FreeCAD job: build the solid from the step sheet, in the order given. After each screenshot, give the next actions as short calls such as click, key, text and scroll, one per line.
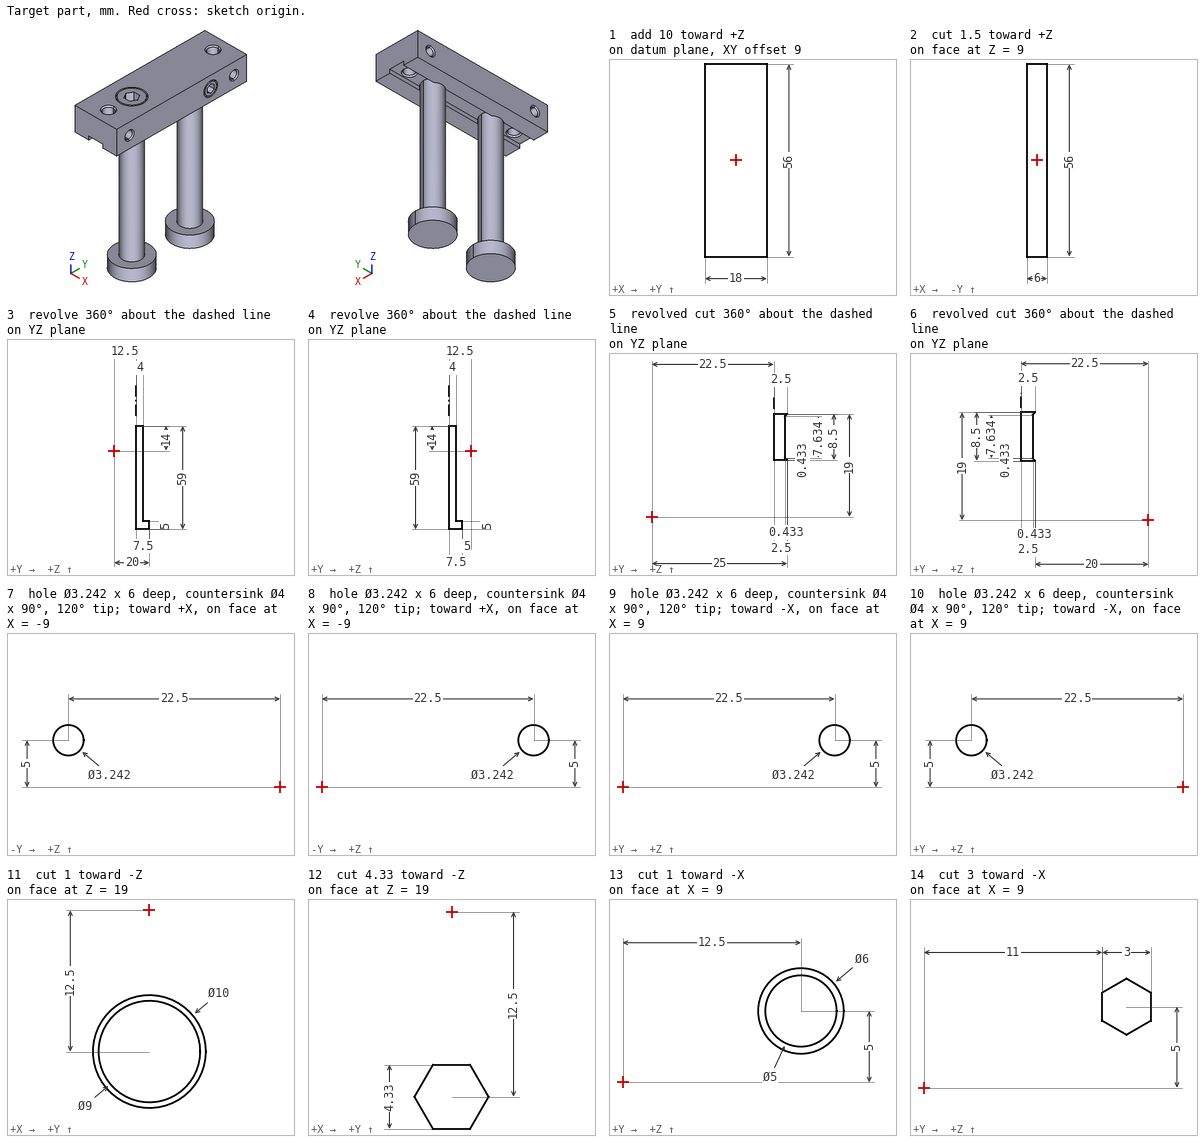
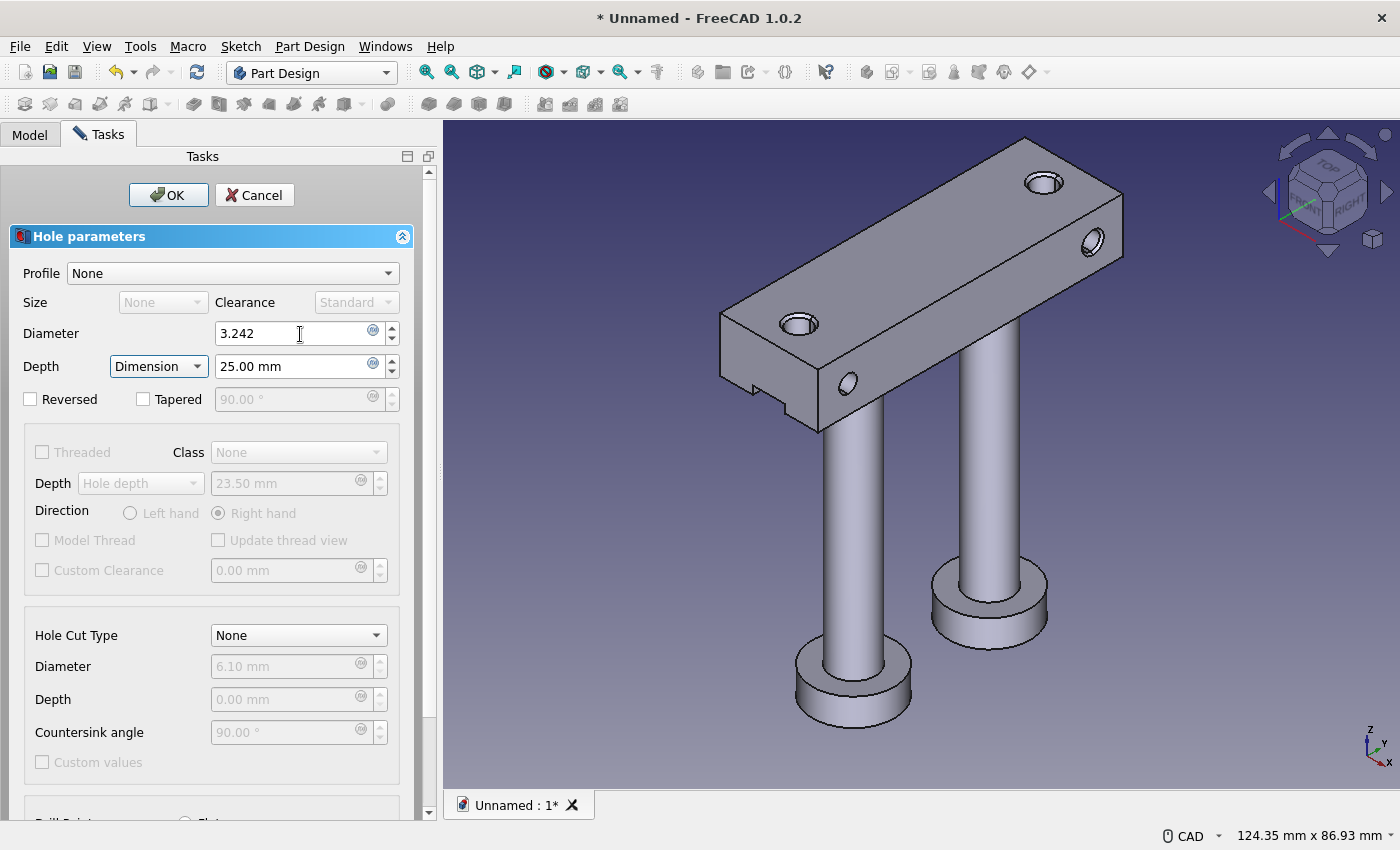
triple_click(300, 366)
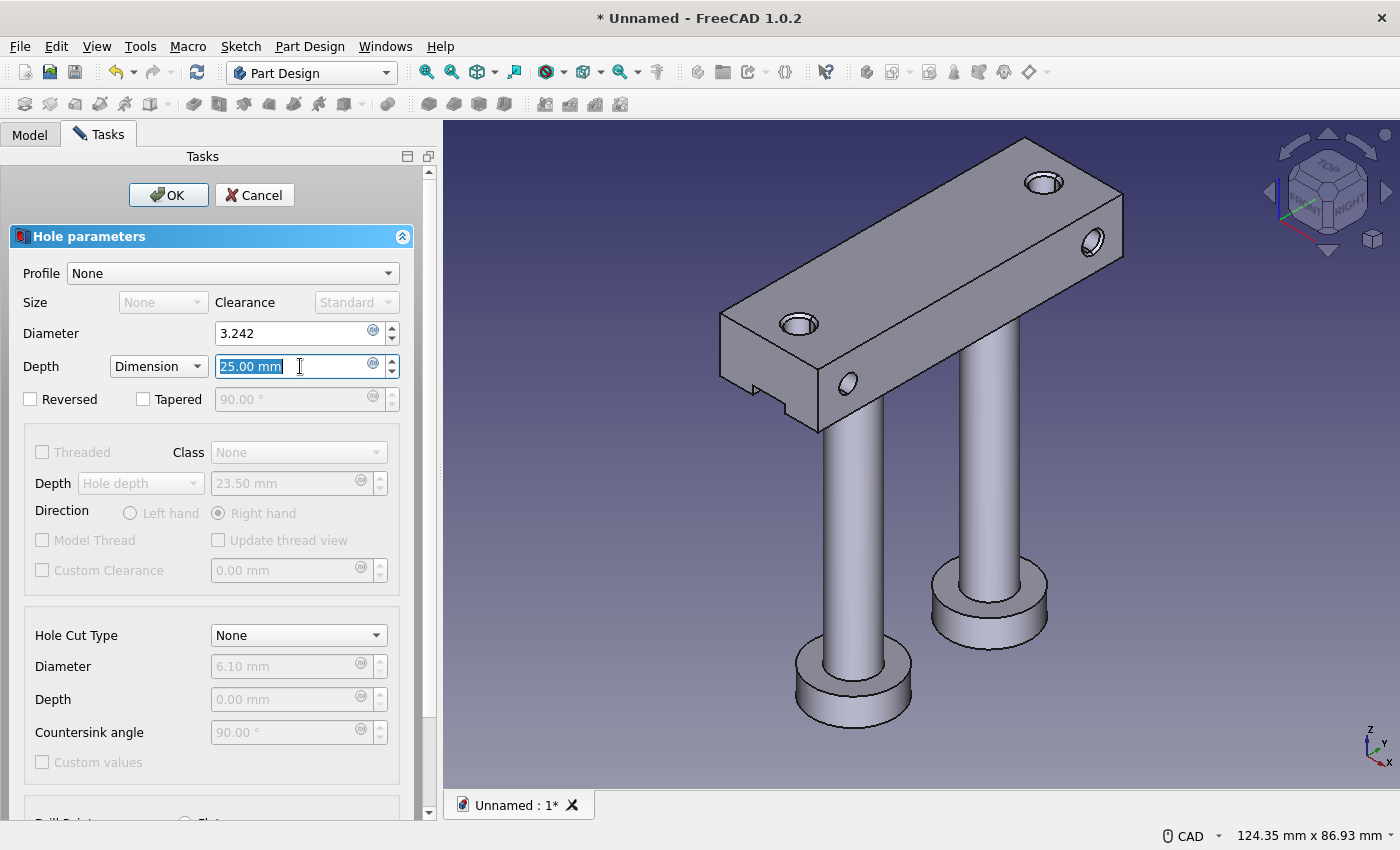
text(6)
key(Tab)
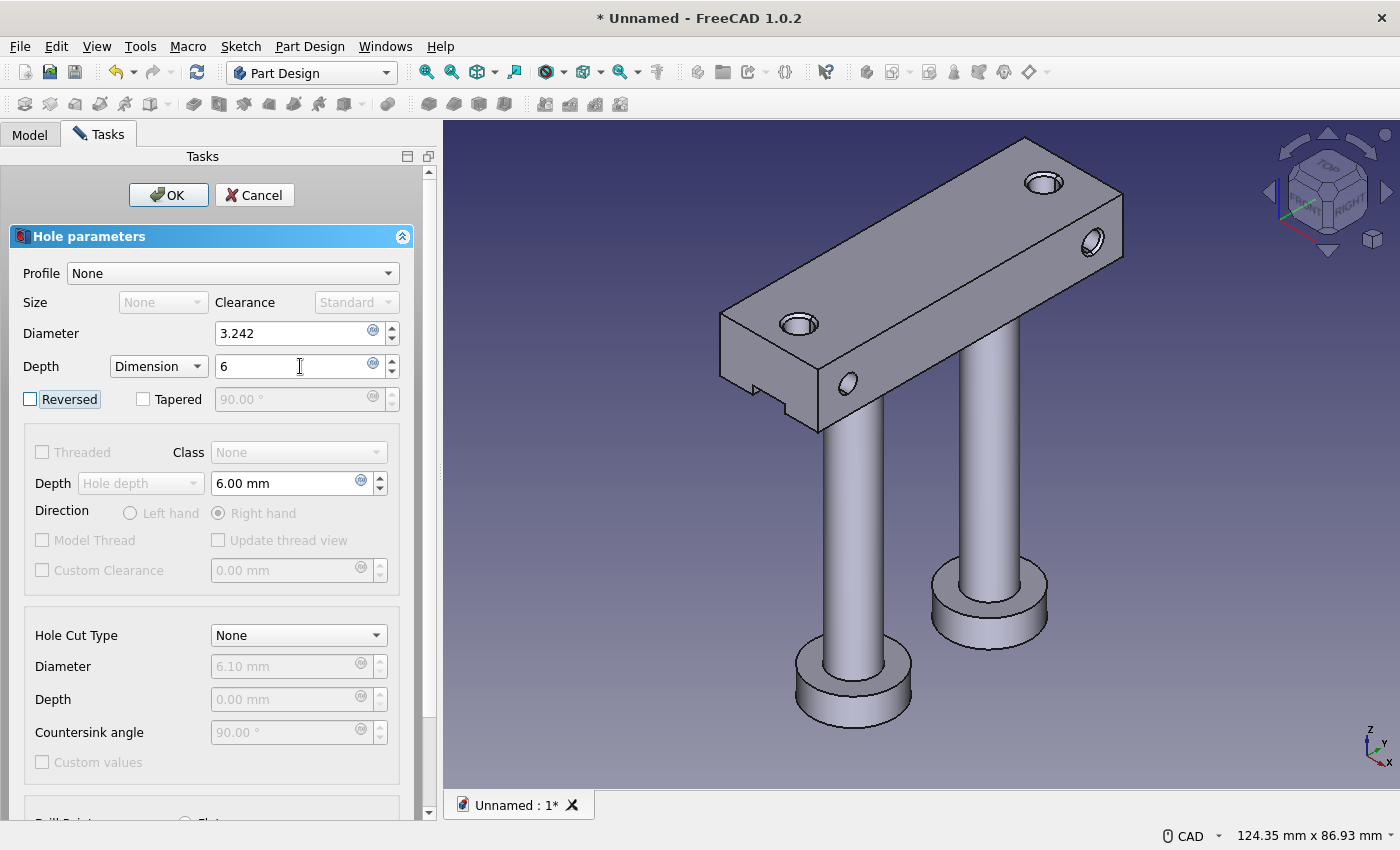
click(300, 636)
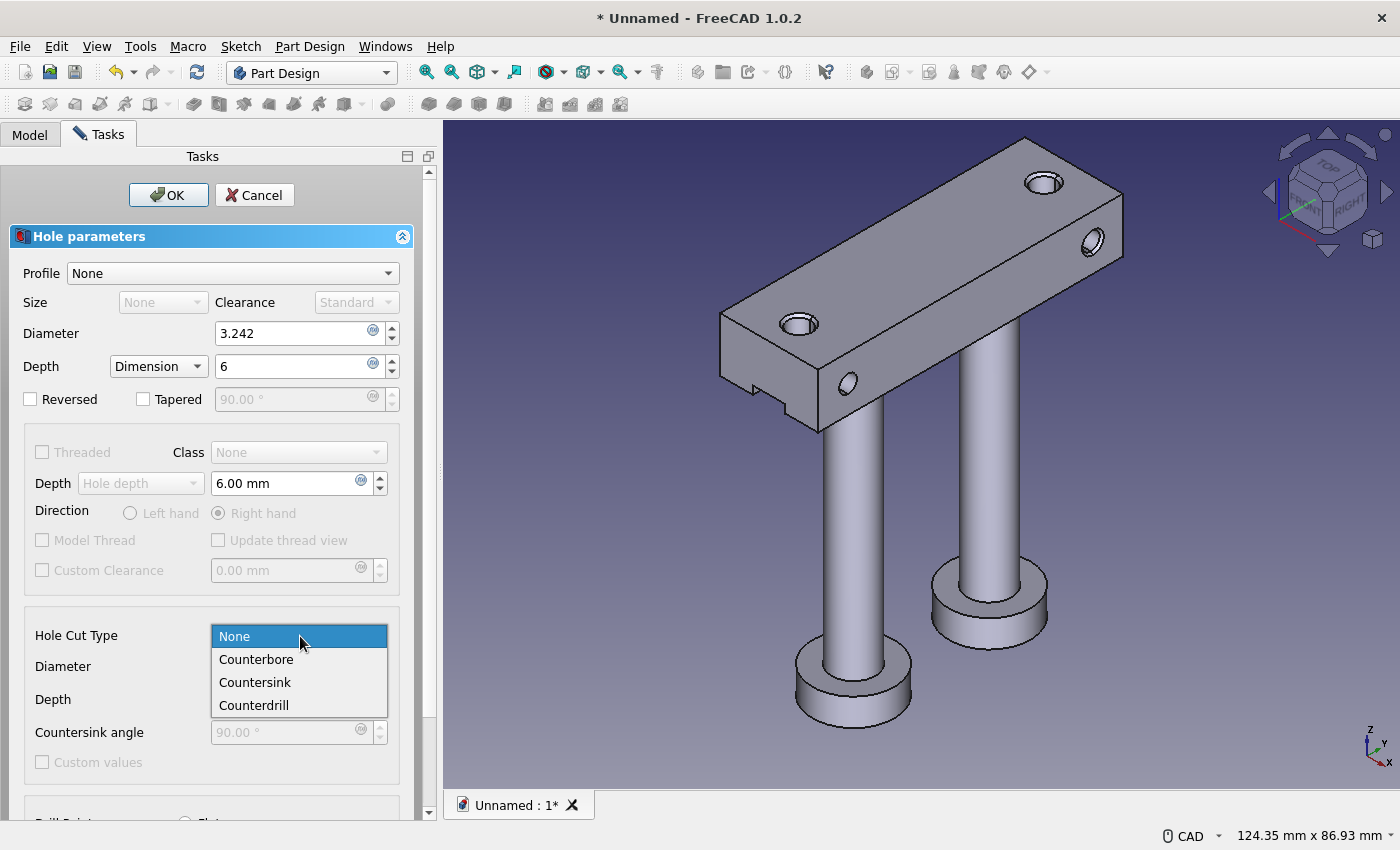
click(298, 682)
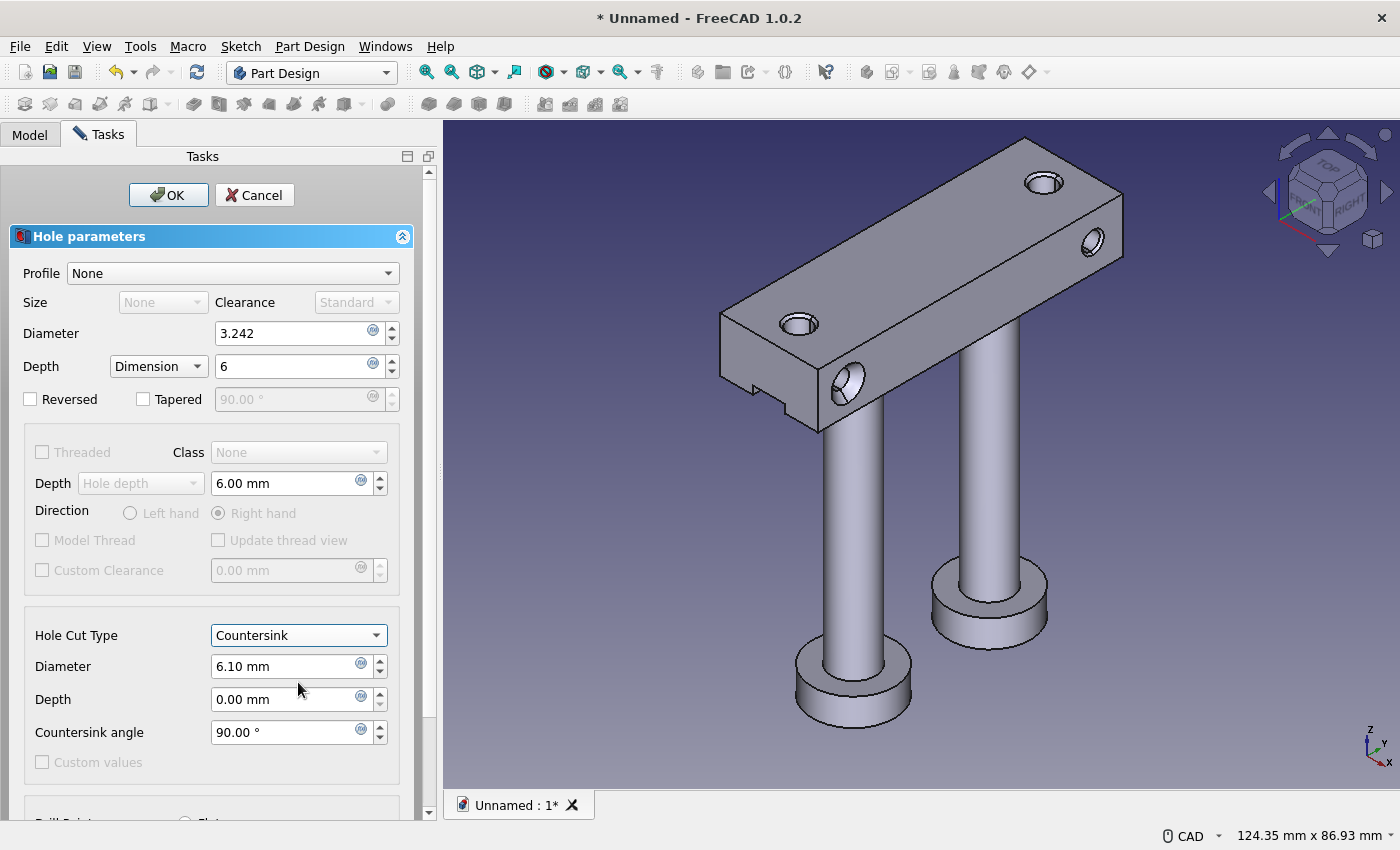
triple_click(292, 666)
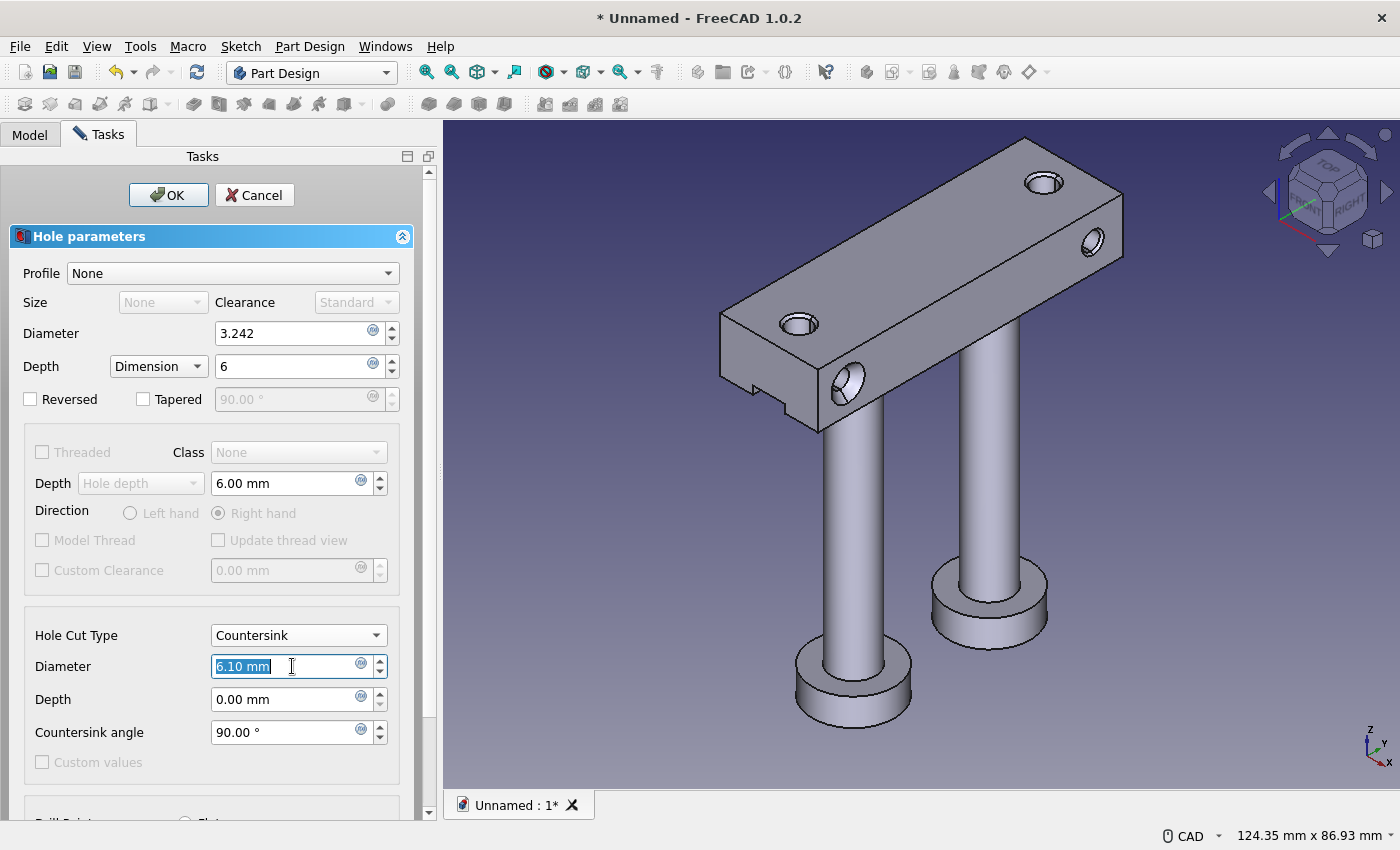
text(4)
key(Tab)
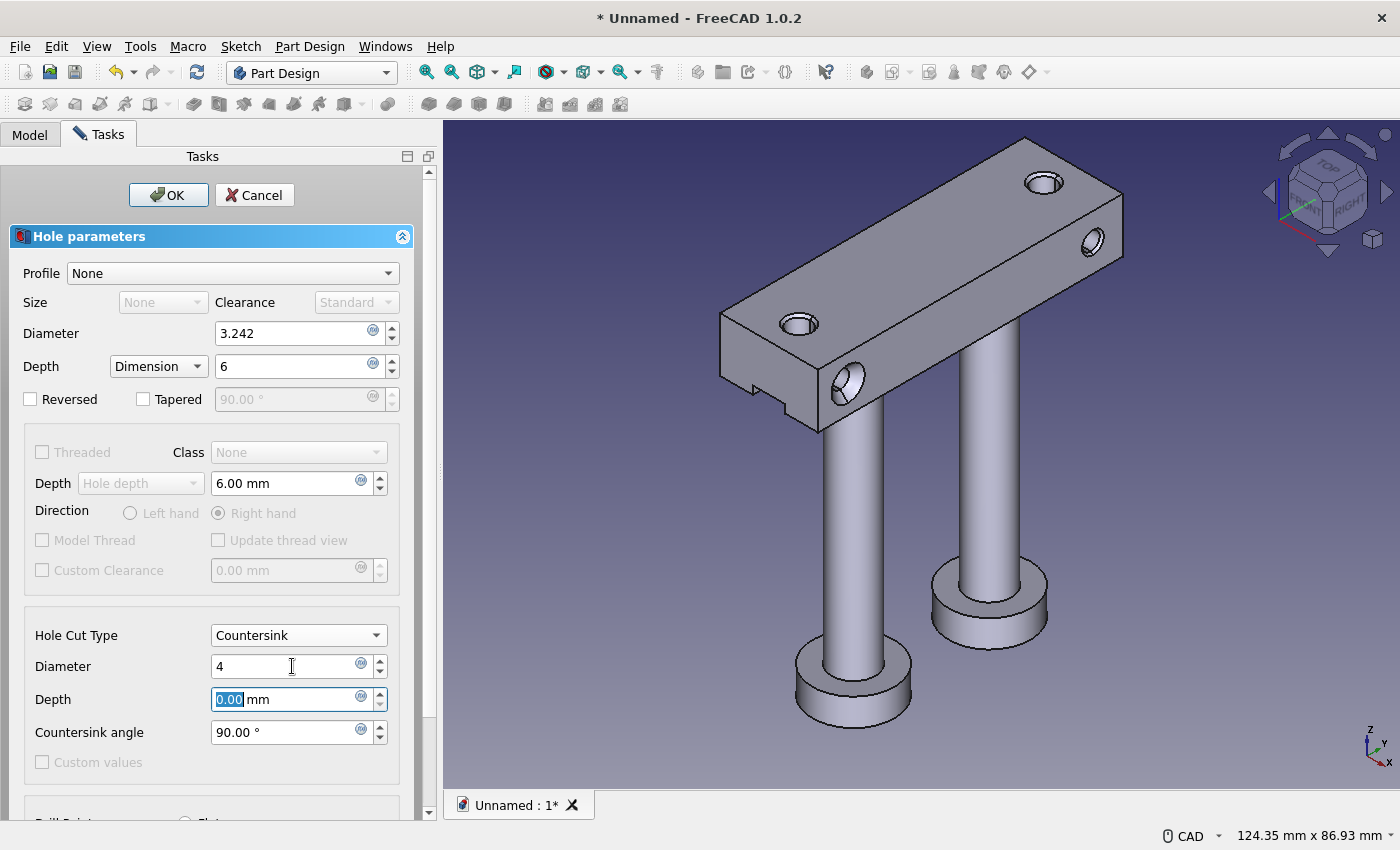
scroll(429, 493, down, 2)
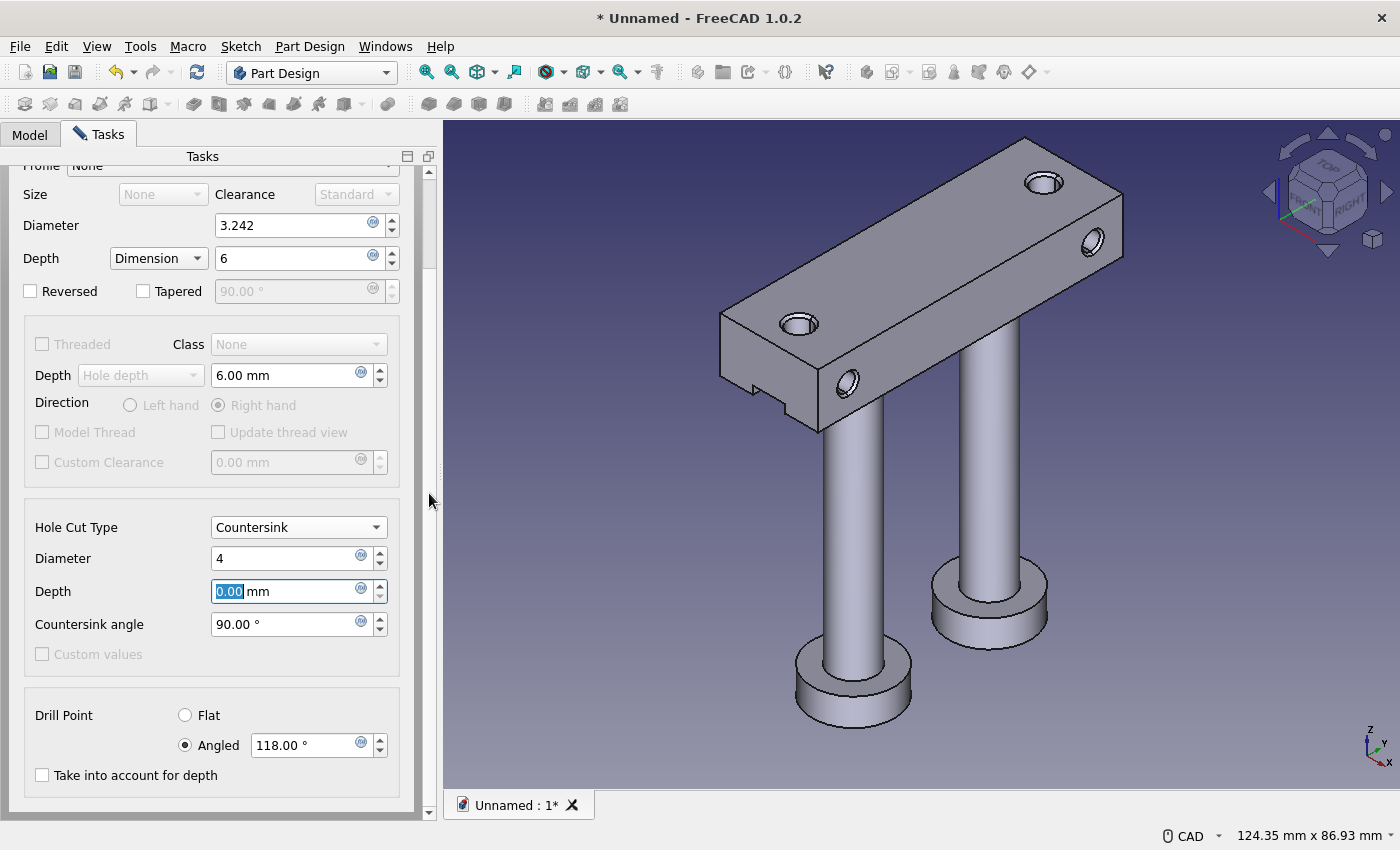
triple_click(312, 746)